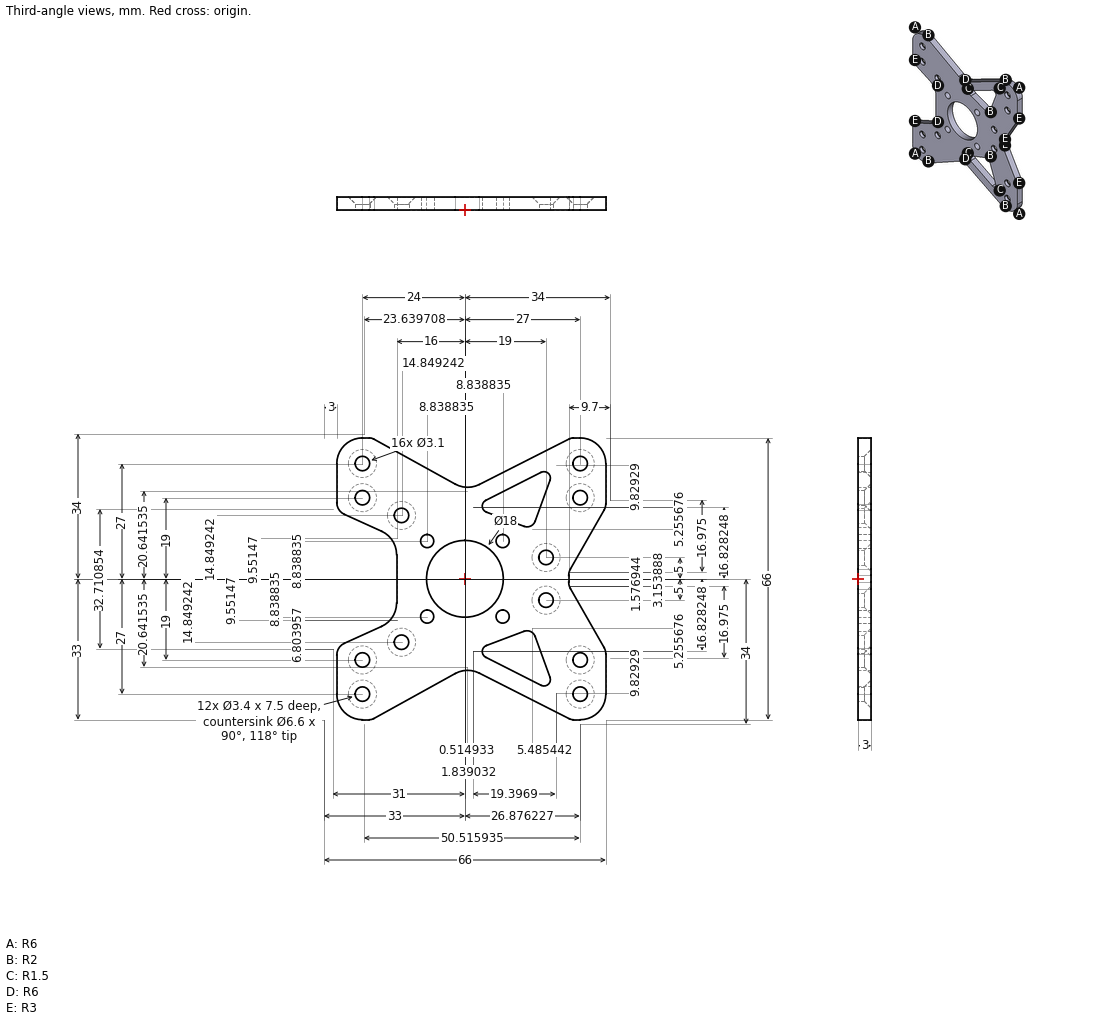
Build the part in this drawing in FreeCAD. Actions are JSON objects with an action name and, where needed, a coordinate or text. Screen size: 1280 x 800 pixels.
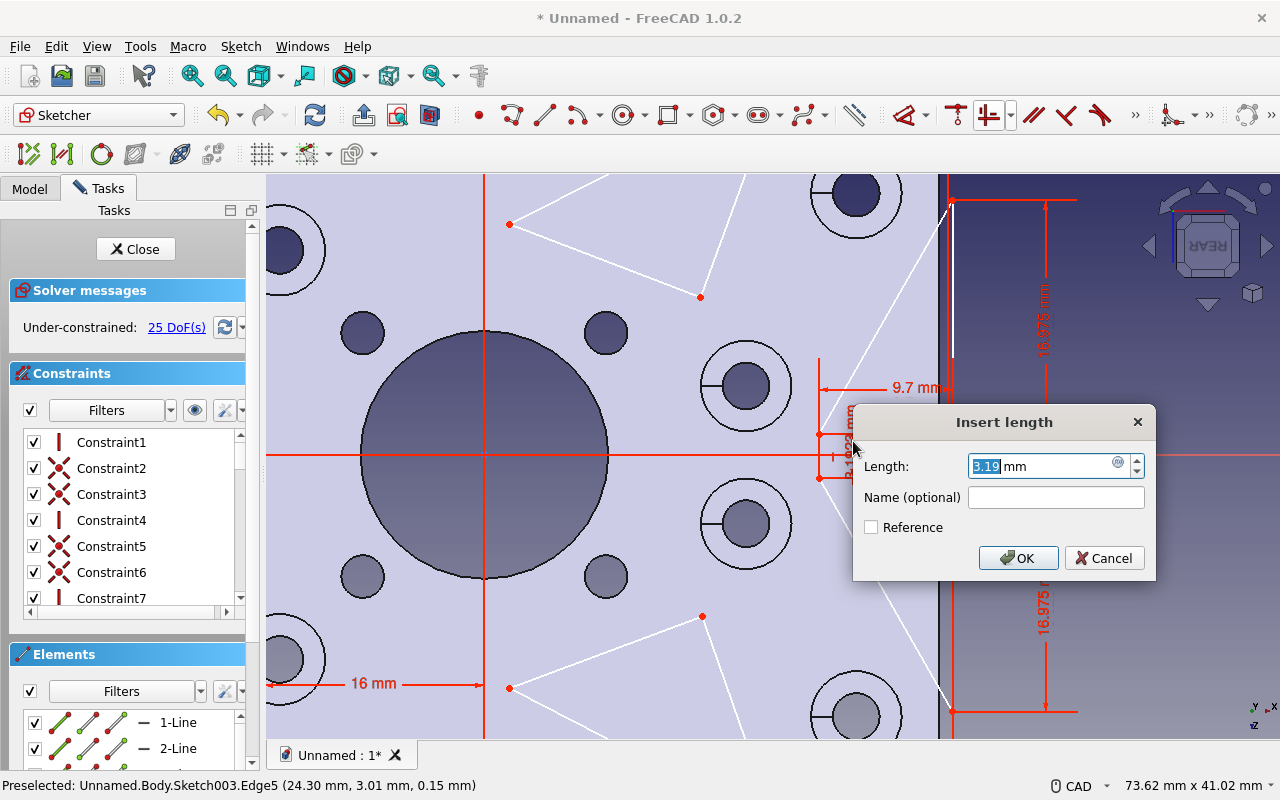
{"action": "type", "text": "3.153888"}
{"action": "key", "text": "Return"}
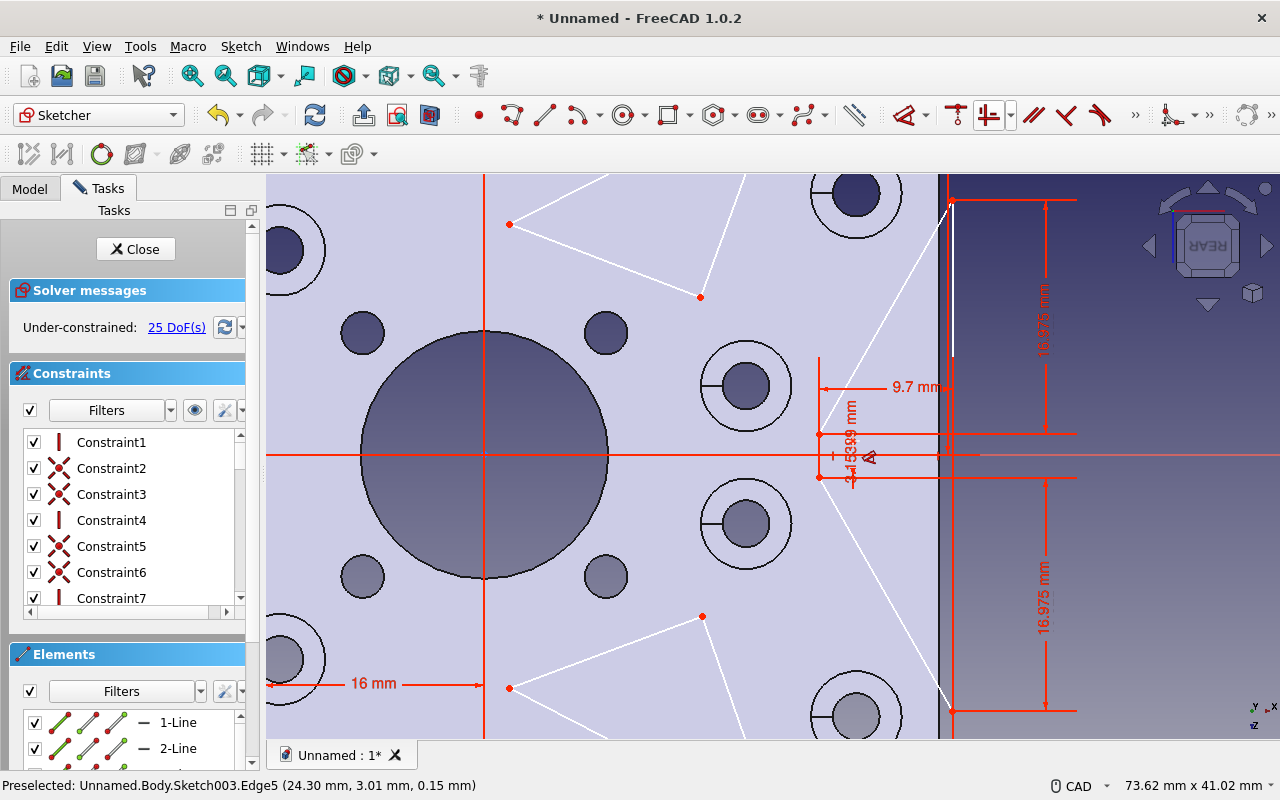
{"action": "scroll", "coordinate": [821, 457], "scroll_direction": "down", "scroll_amount": 5}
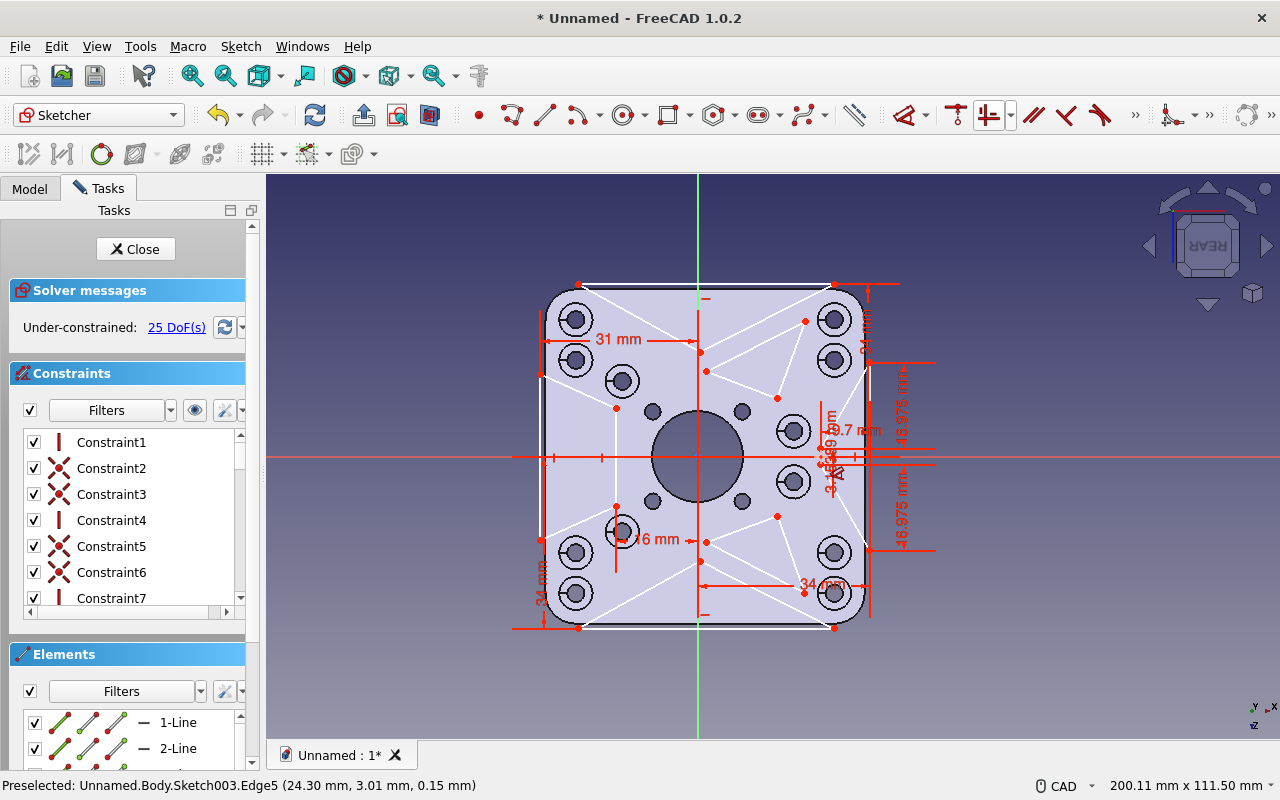
{"action": "left_click", "coordinate": [616, 506]}
{"action": "left_click", "coordinate": [582, 481]}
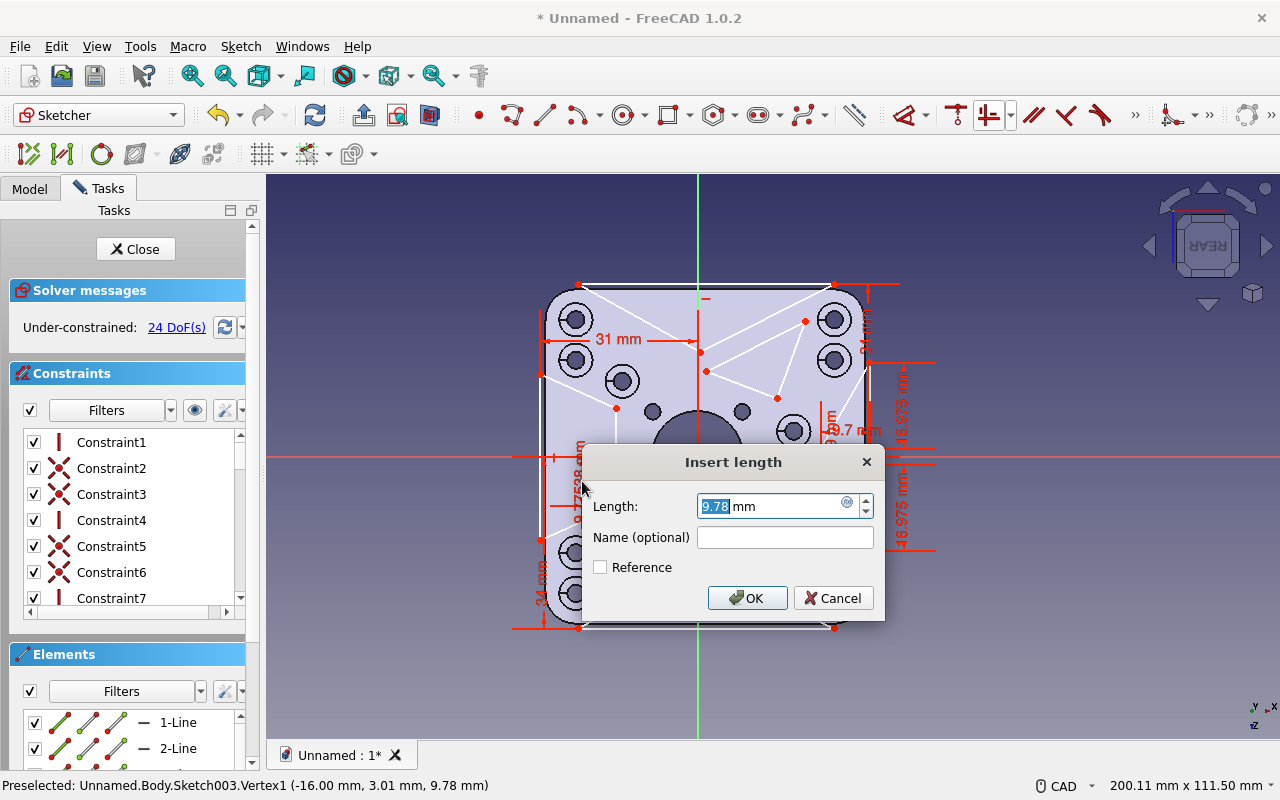
{"action": "type", "text": "9.55147"}
{"action": "key", "text": "Return"}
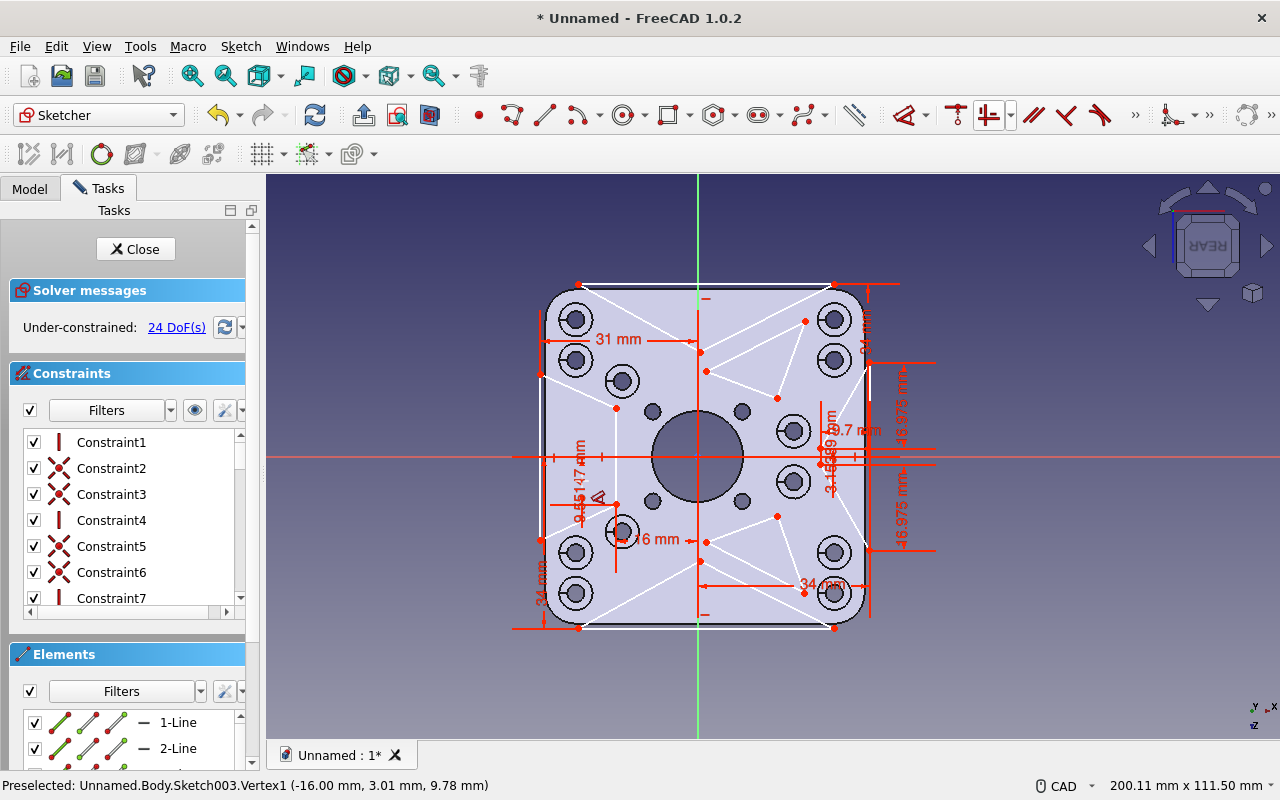
{"action": "left_click", "coordinate": [616, 409]}
{"action": "left_click", "coordinate": [582, 433]}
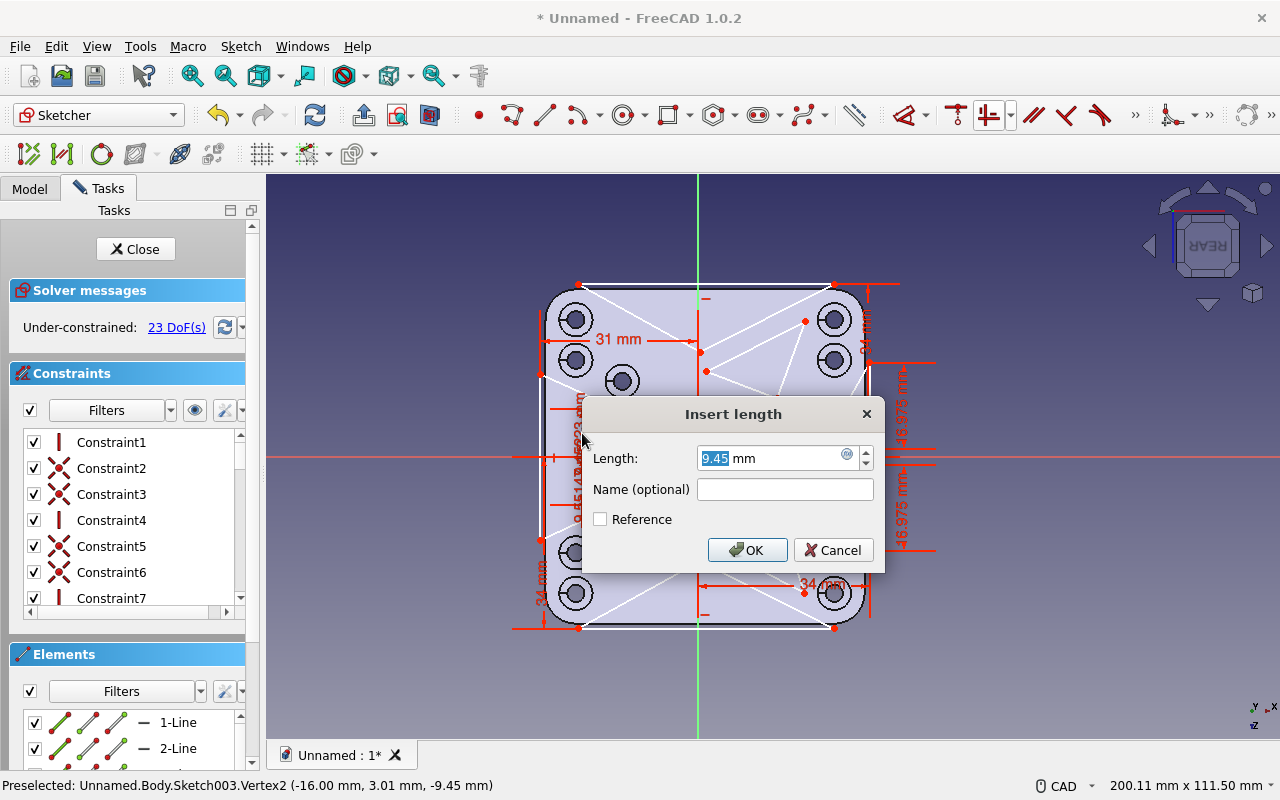
{"action": "type", "text": "9.55147"}
{"action": "key", "text": "Return"}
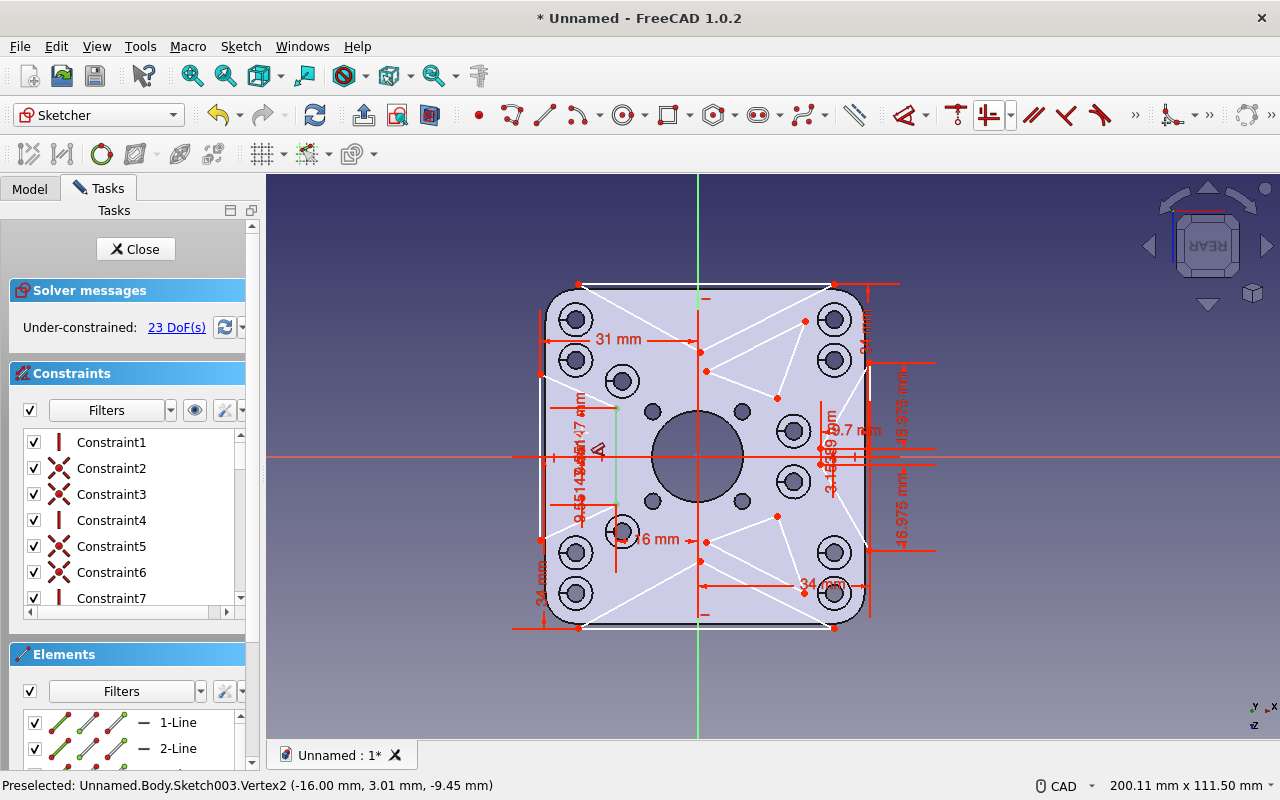
{"action": "left_click", "coordinate": [776, 337]}
{"action": "left_click", "coordinate": [756, 406]}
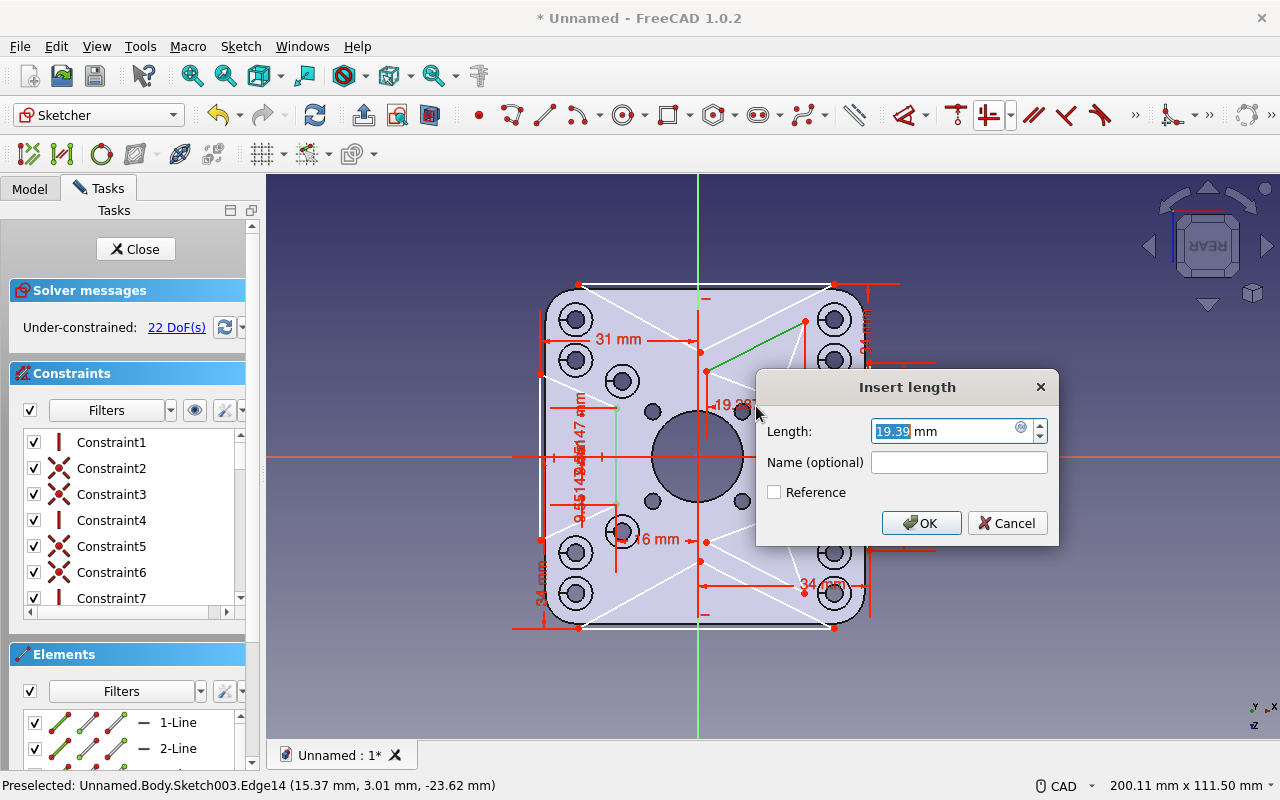
{"action": "type", "text": "19.3969"}
{"action": "key", "text": "Return"}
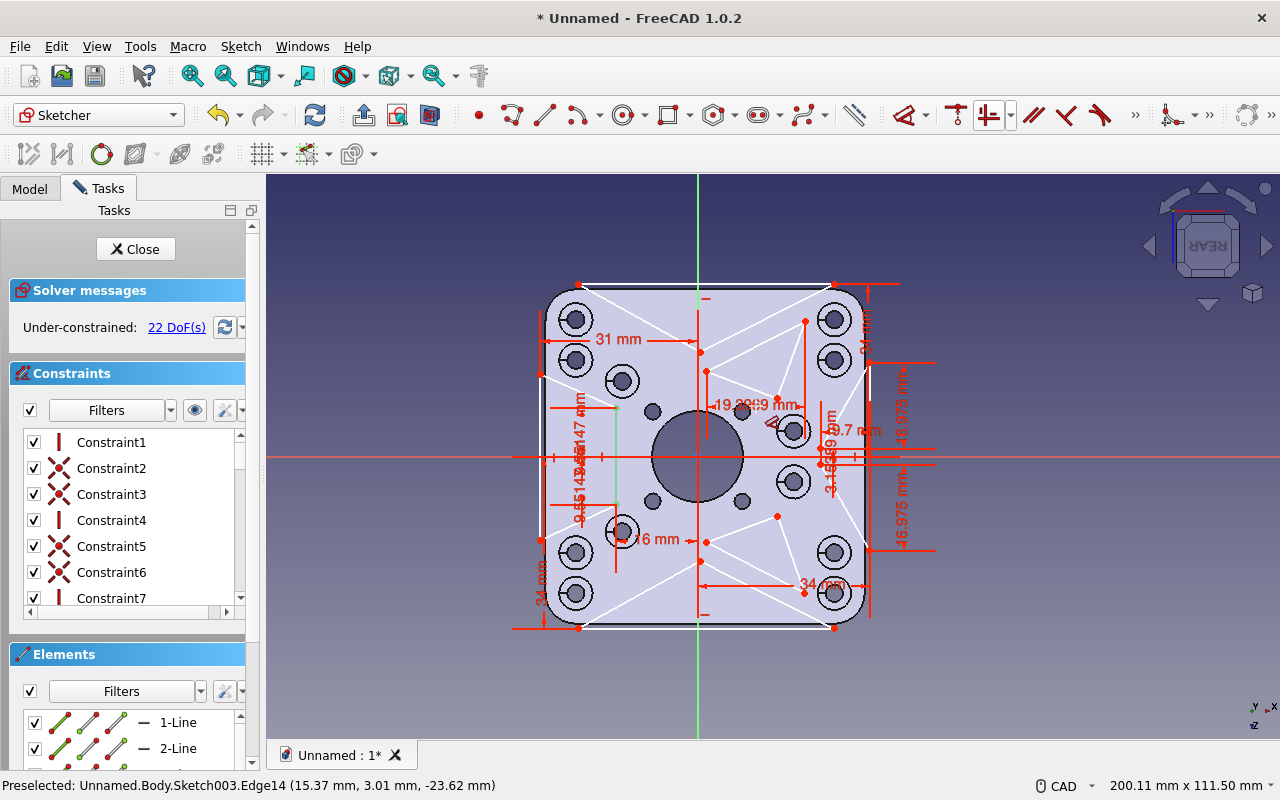
{"action": "left_click", "coordinate": [776, 337]}
{"action": "left_click", "coordinate": [839, 358]}